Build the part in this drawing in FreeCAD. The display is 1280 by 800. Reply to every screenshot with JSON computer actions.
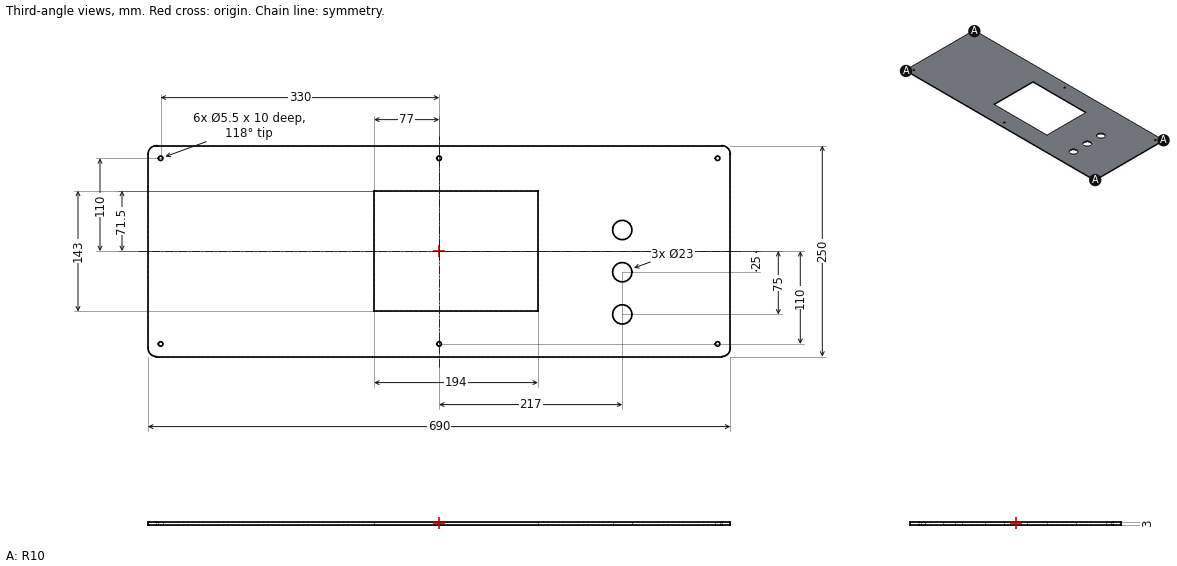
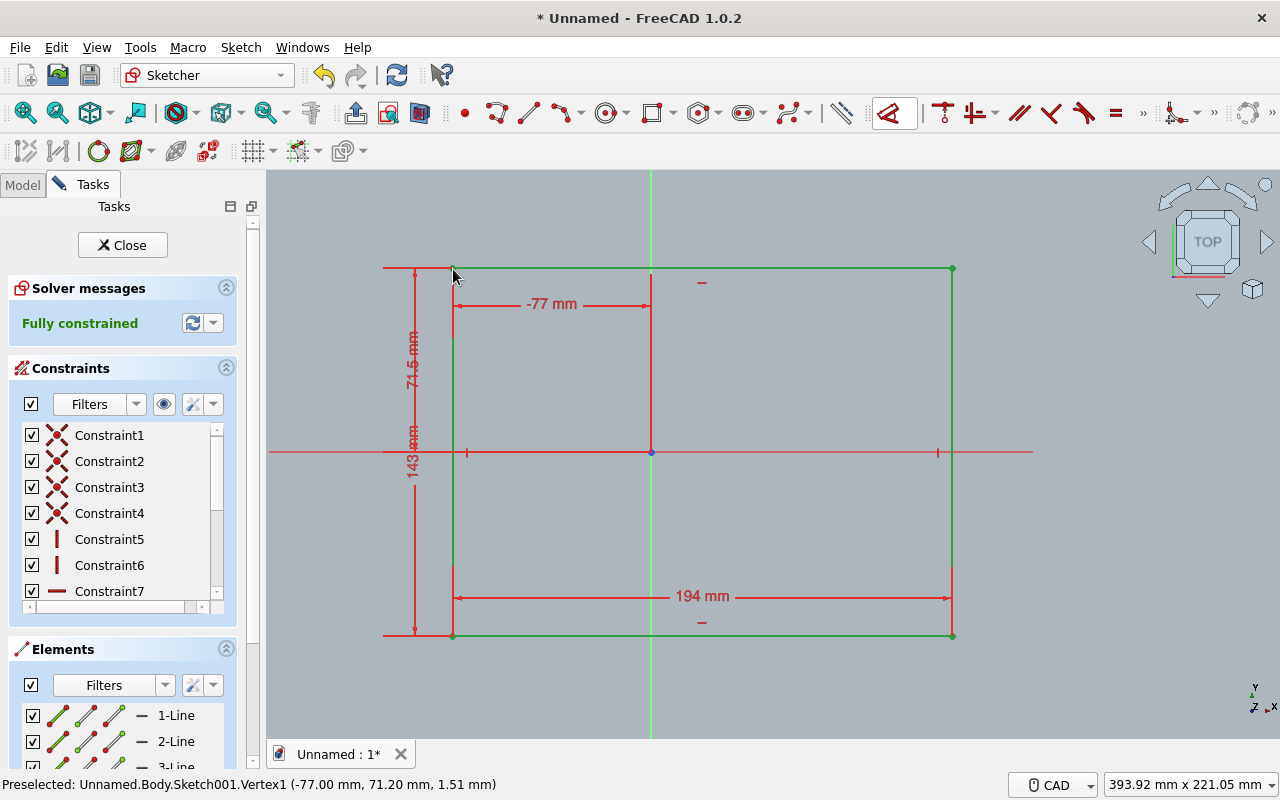
{"action": "left_click", "coordinate": [123, 245]}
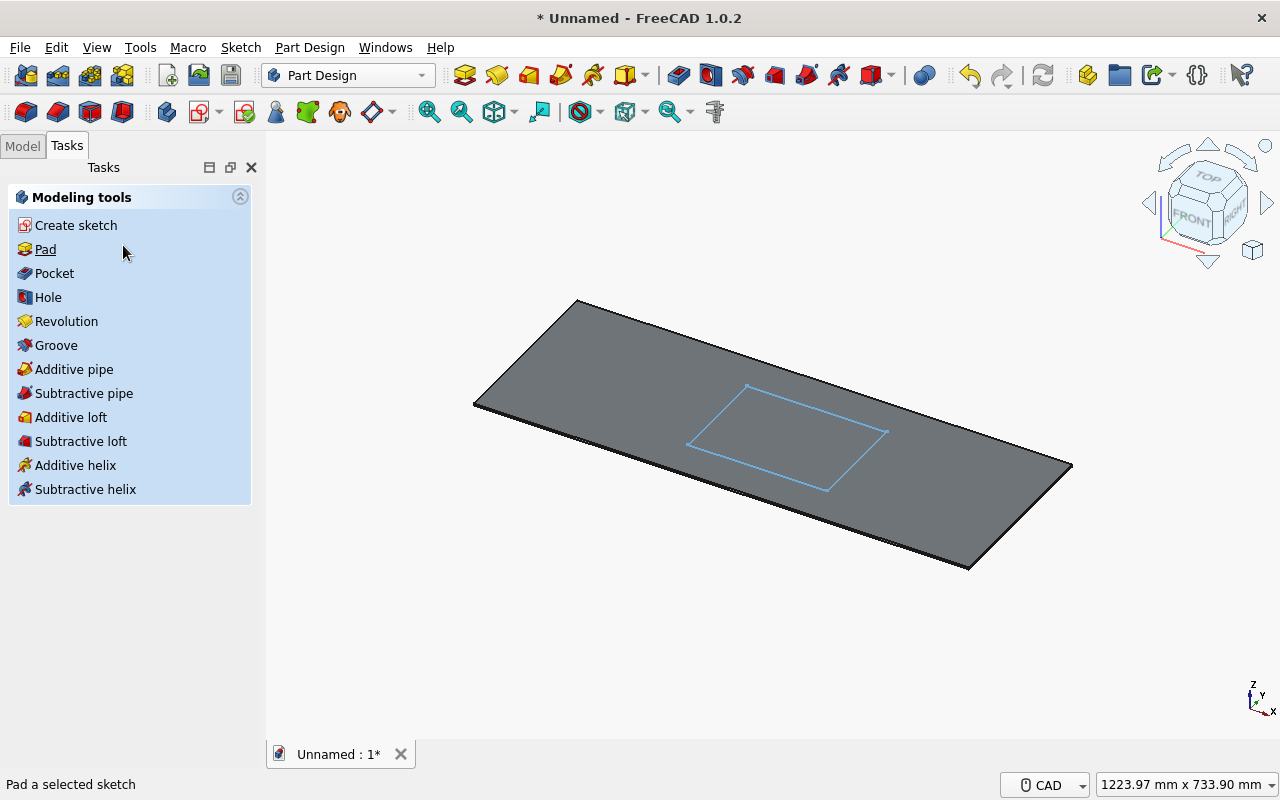
{"action": "left_click", "coordinate": [680, 76]}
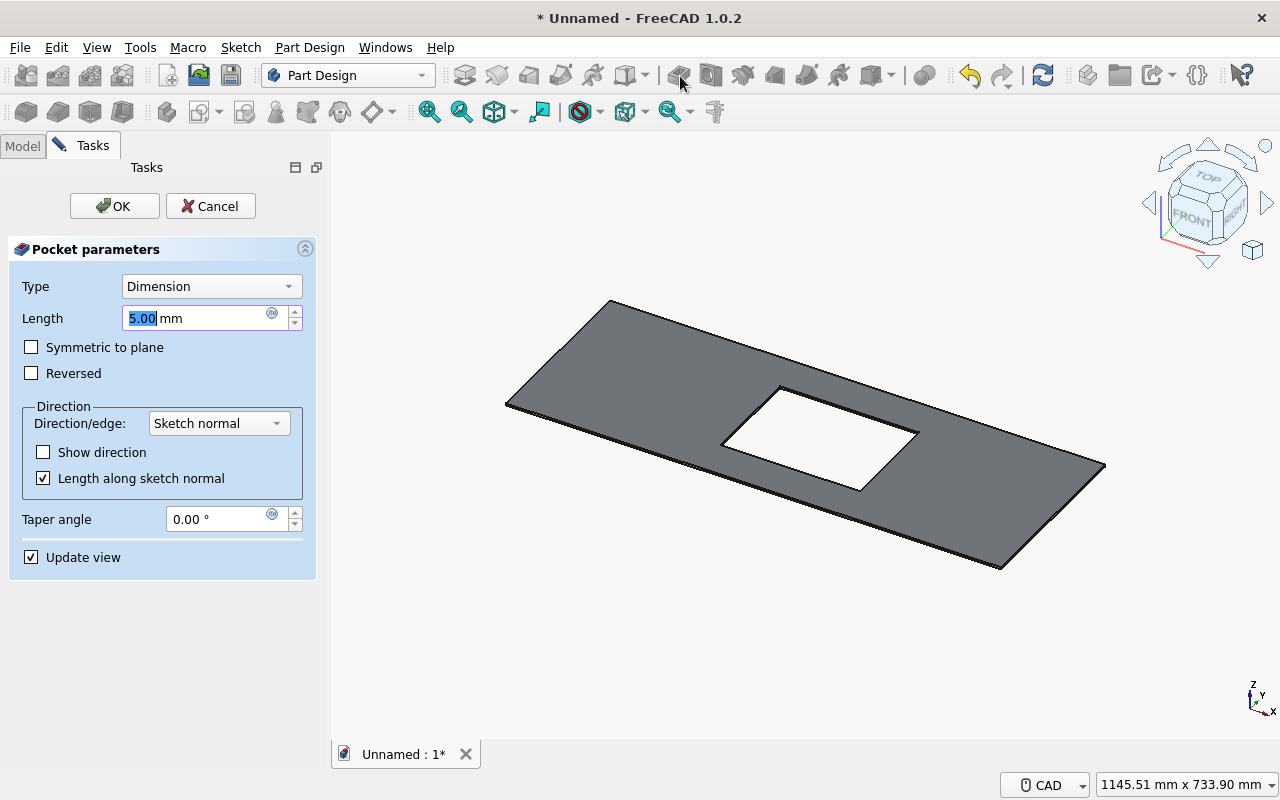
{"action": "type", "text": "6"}
{"action": "key", "text": "Tab"}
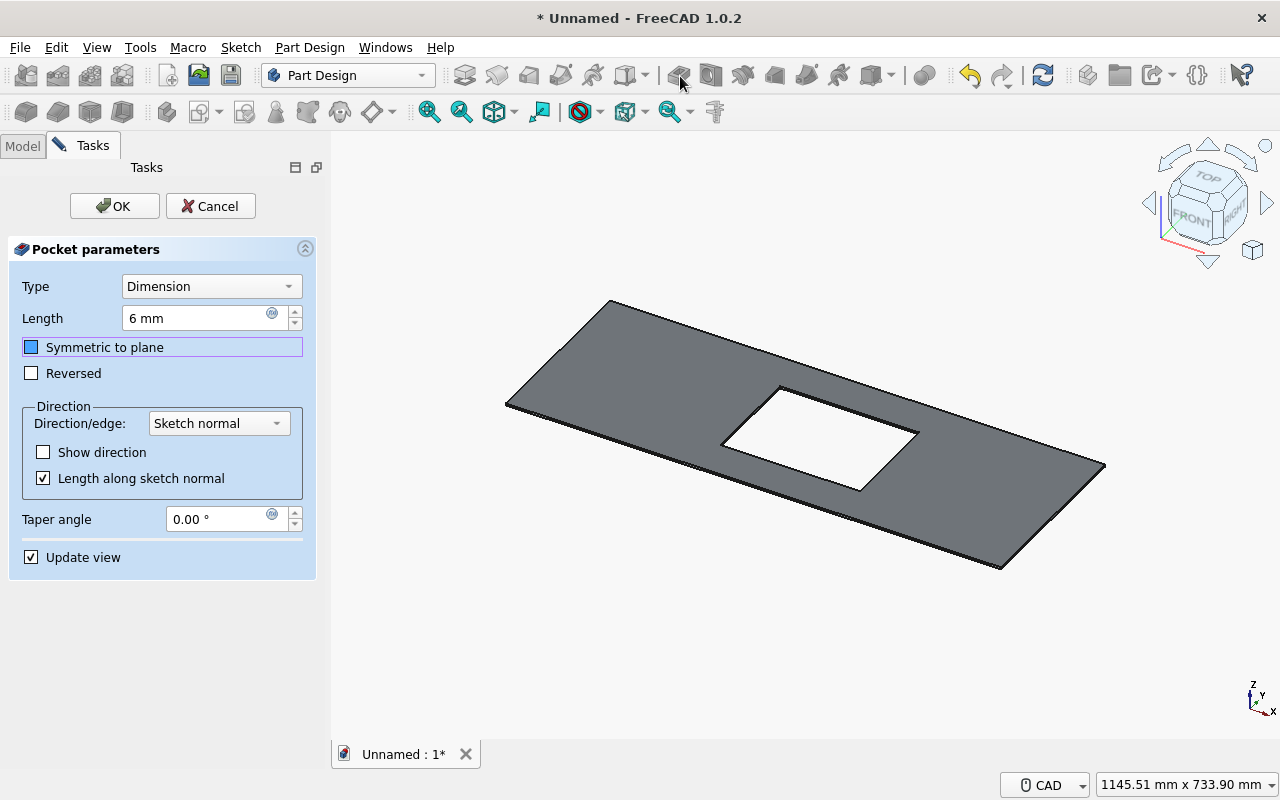
{"action": "left_click", "coordinate": [115, 206]}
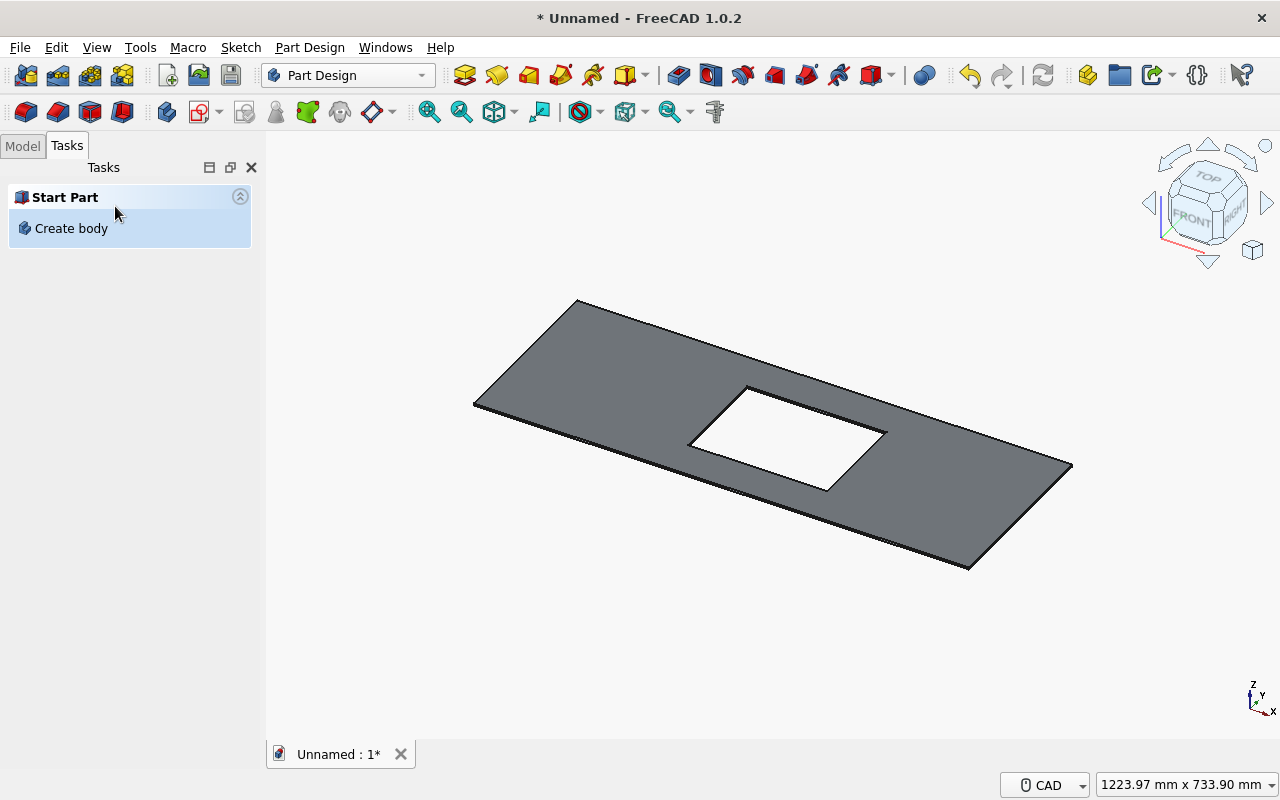
{"action": "left_click", "coordinate": [632, 386]}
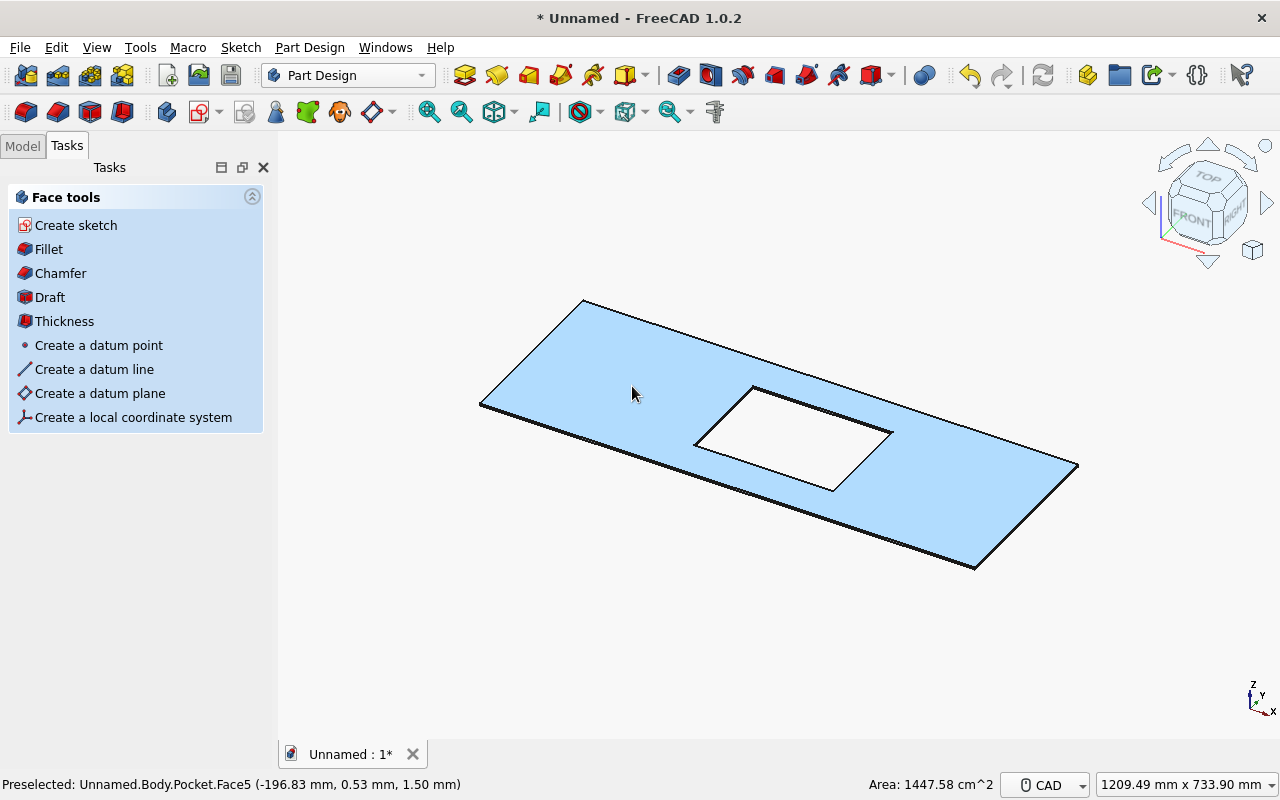
{"action": "left_click", "coordinate": [200, 112]}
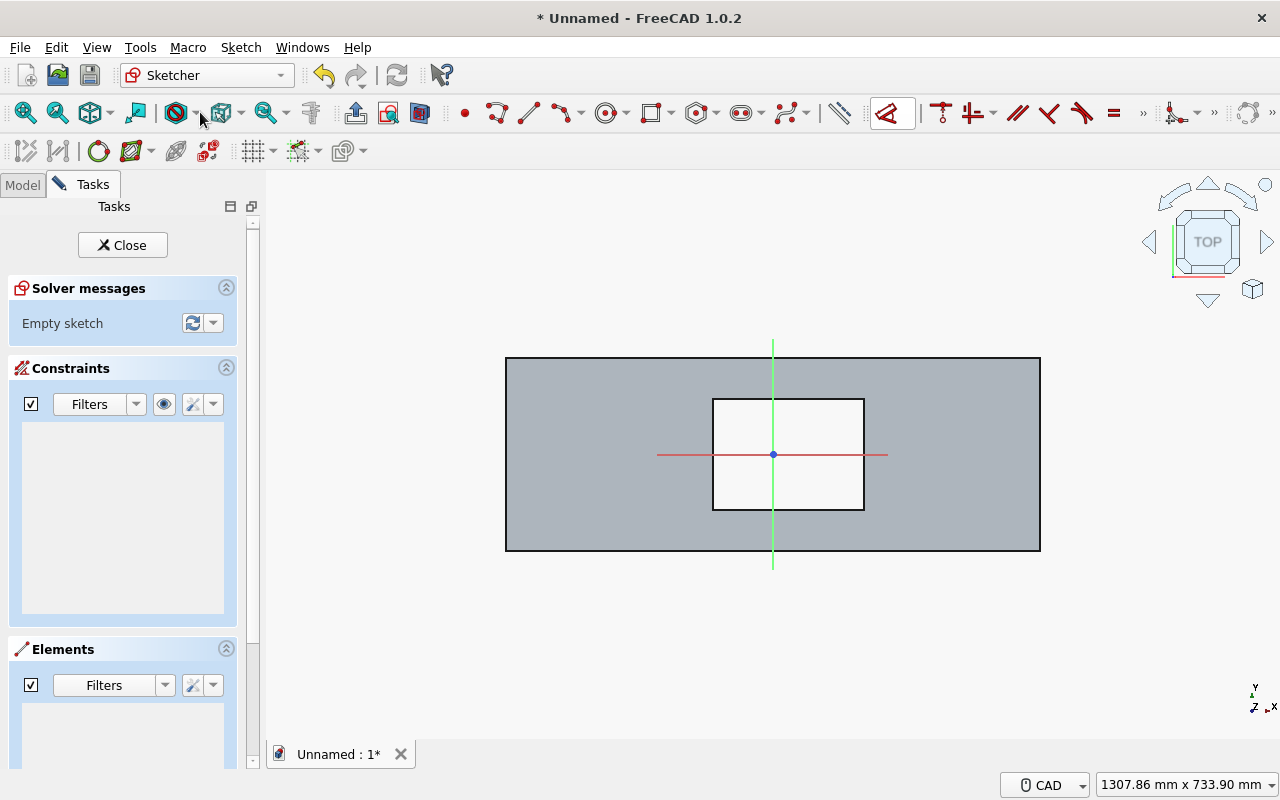
{"action": "scroll", "coordinate": [929, 482], "scroll_direction": "up", "scroll_amount": 6}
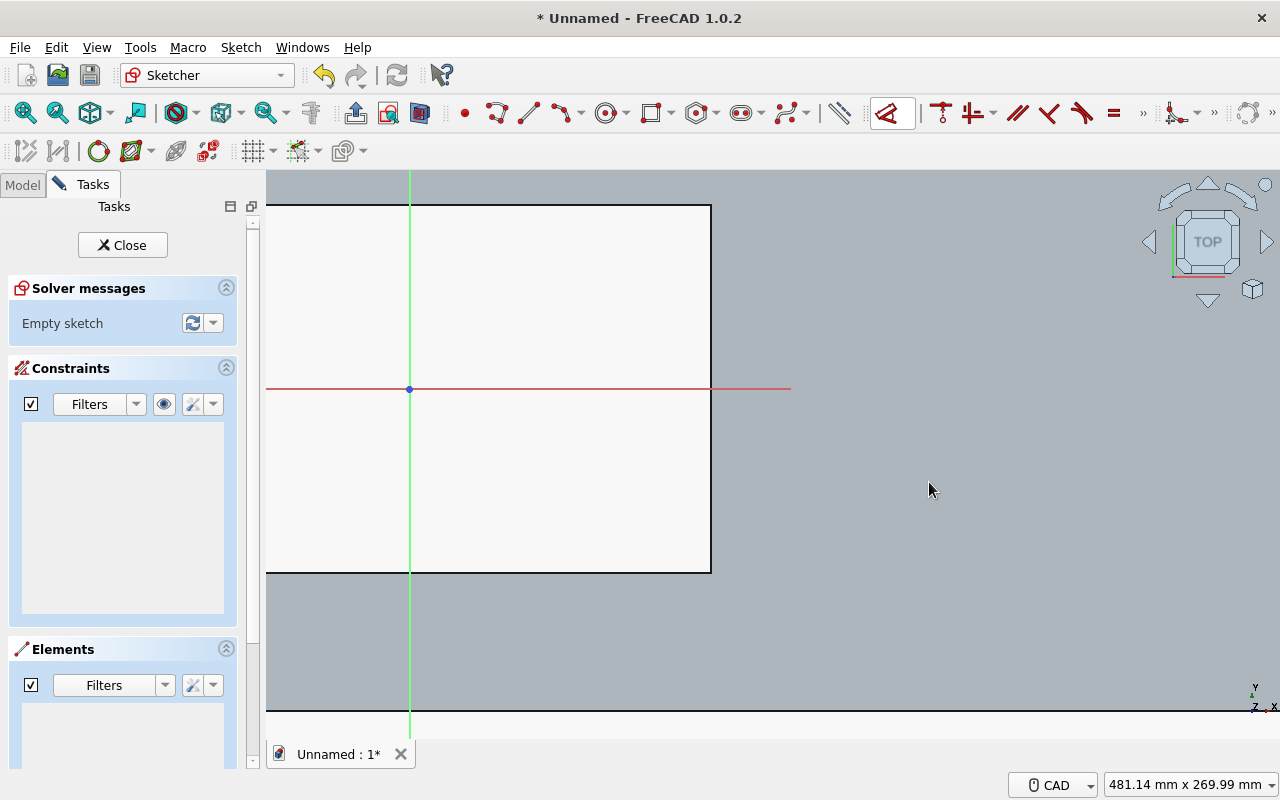
{"action": "left_click", "coordinate": [606, 114]}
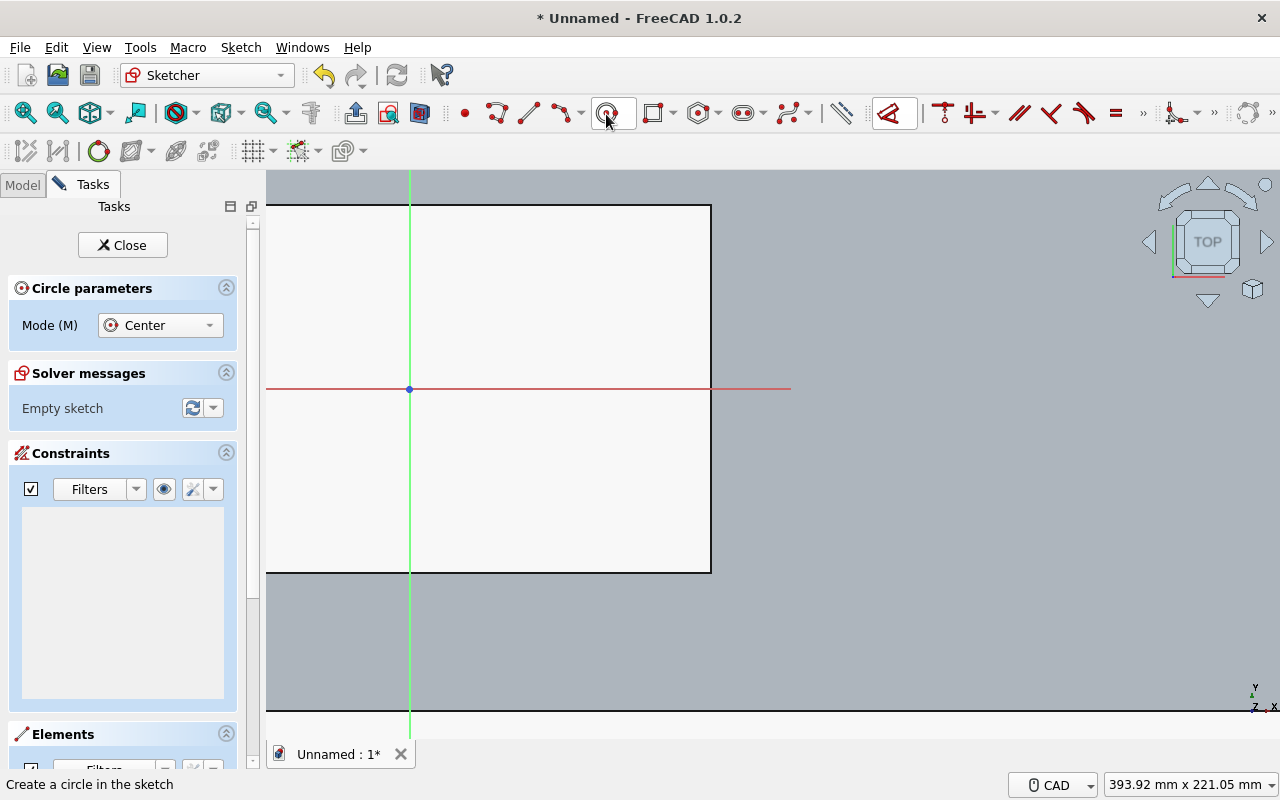
{"action": "left_click", "coordinate": [968, 454]}
{"action": "left_click", "coordinate": [989, 433]}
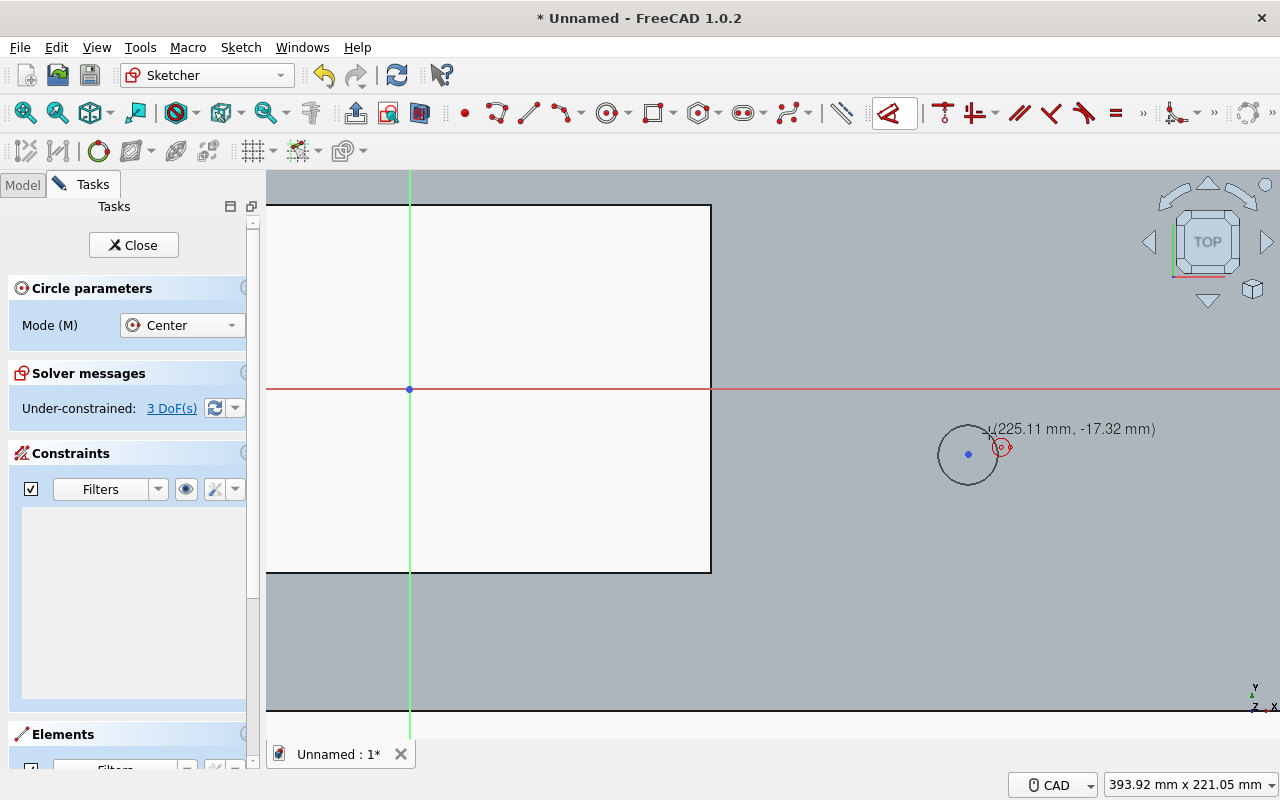
{"action": "left_click", "coordinate": [968, 582]}
{"action": "left_click", "coordinate": [989, 562]}